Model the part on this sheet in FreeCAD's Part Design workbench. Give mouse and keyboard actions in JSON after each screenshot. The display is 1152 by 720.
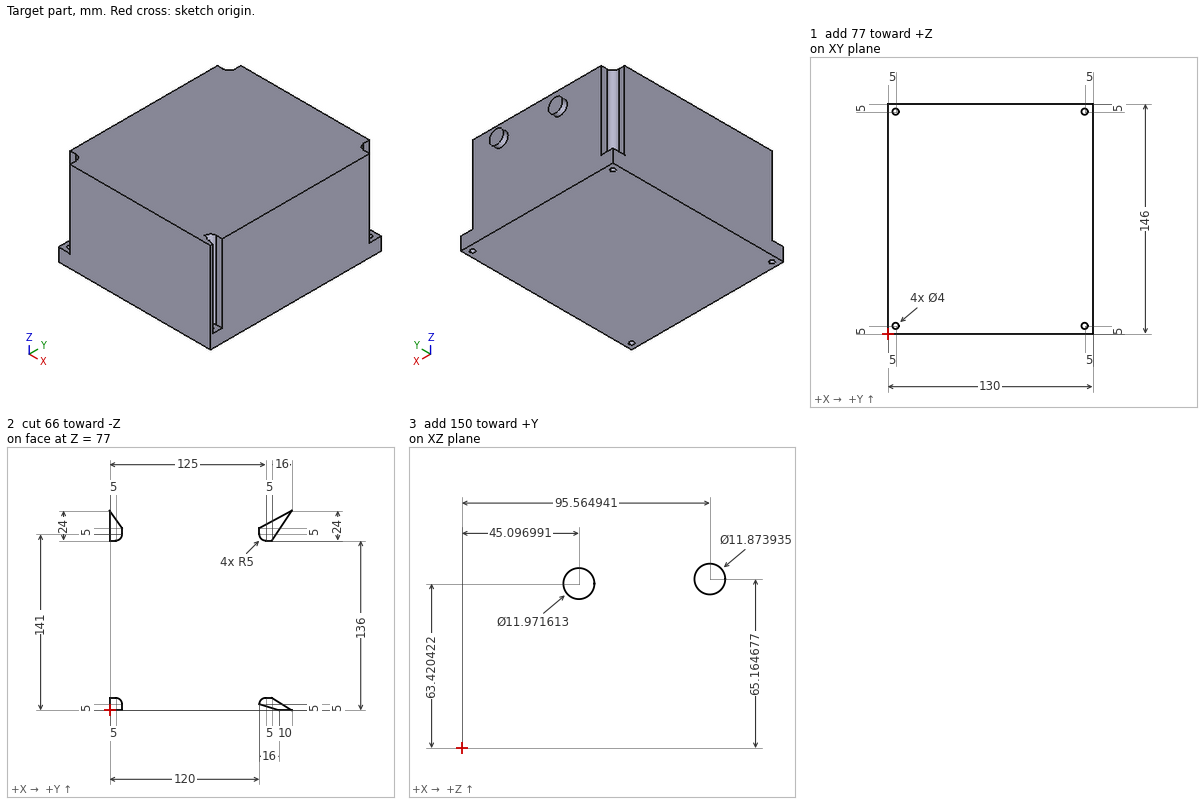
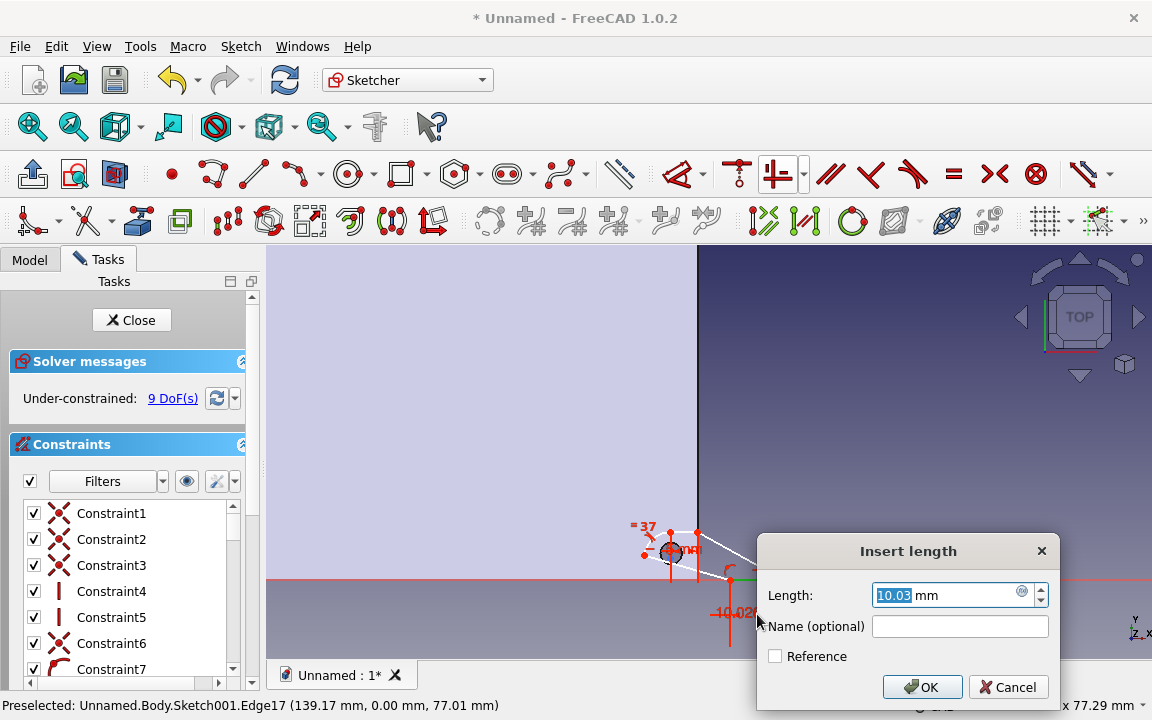
{"action": "type", "text": "10"}
{"action": "key", "text": "Return"}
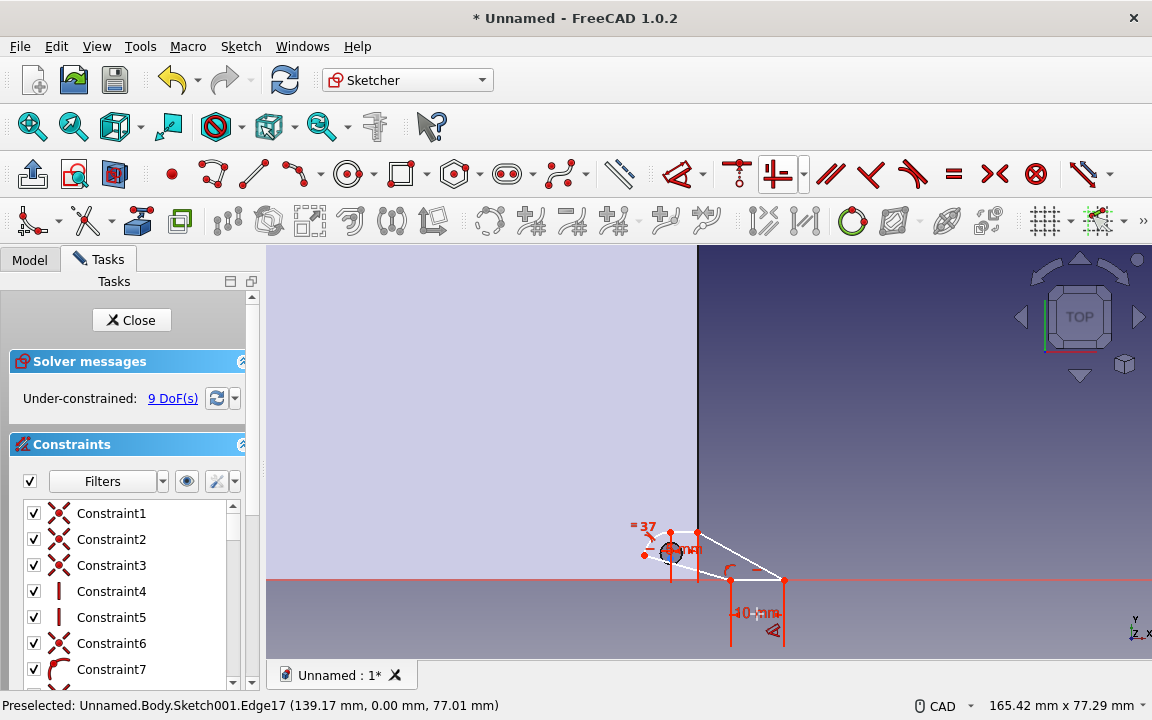
{"action": "scroll", "coordinate": [644, 555], "scroll_direction": "up", "scroll_amount": 2}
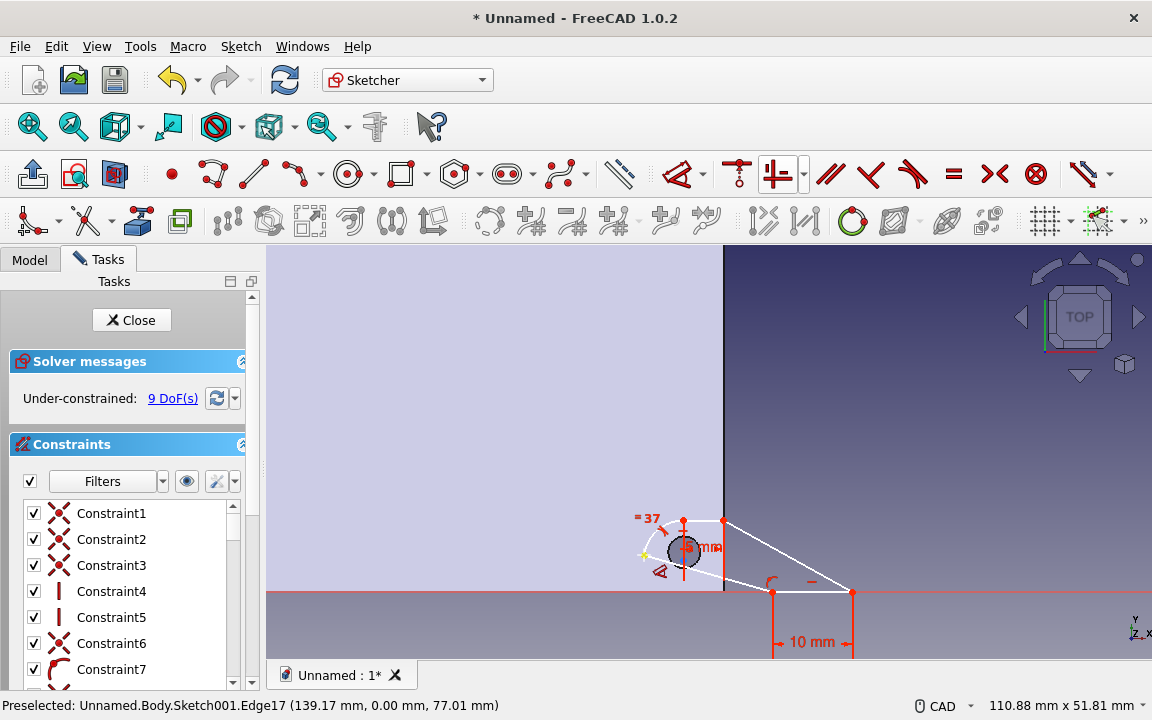
{"action": "left_click", "coordinate": [644, 555]}
{"action": "left_click", "coordinate": [774, 574]}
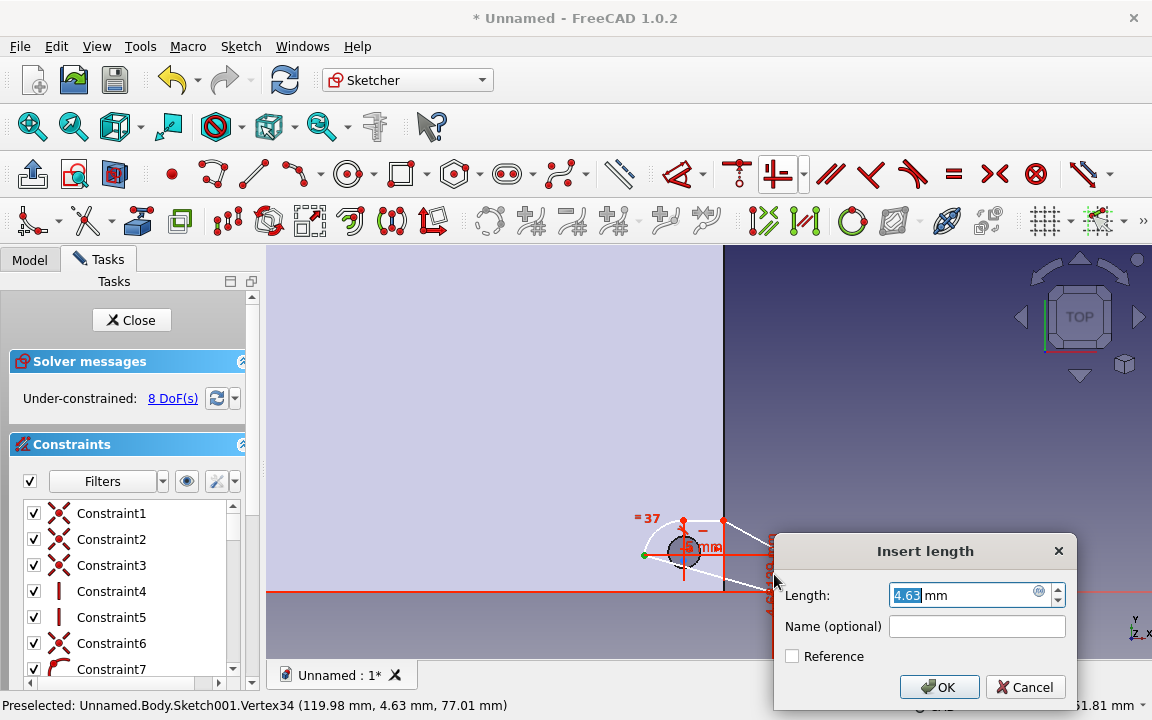
{"action": "type", "text": "5"}
{"action": "key", "text": "Return"}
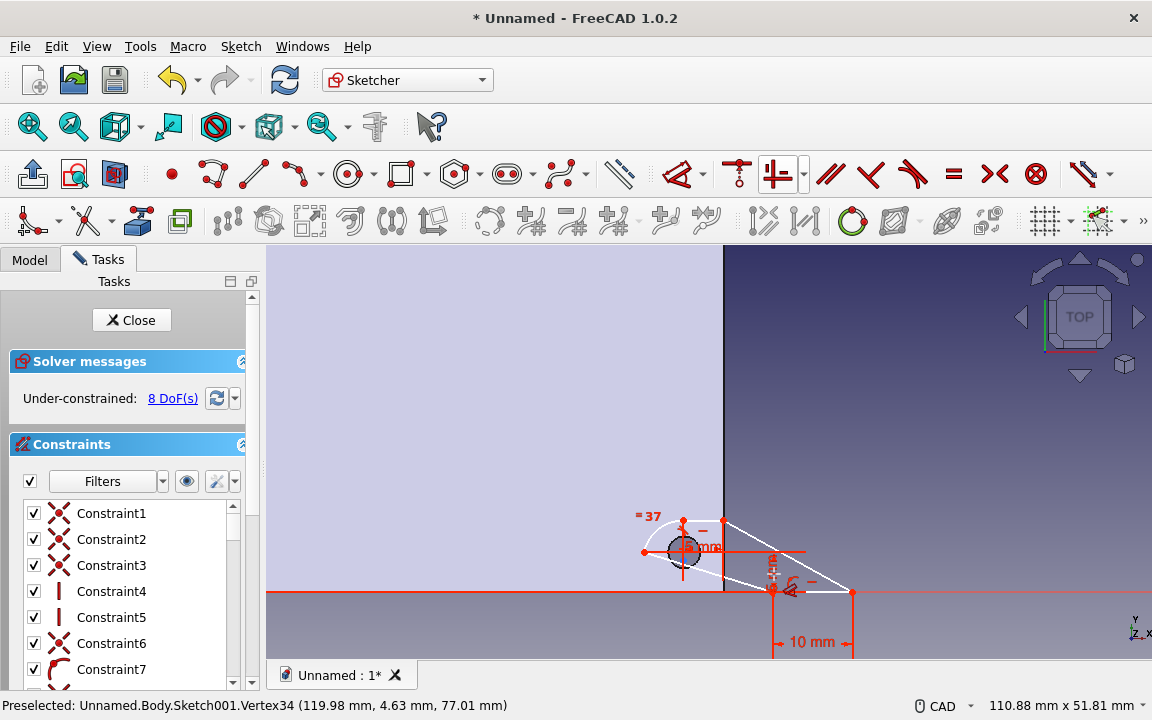
{"action": "left_click", "coordinate": [683, 561]}
{"action": "left_click", "coordinate": [863, 576]}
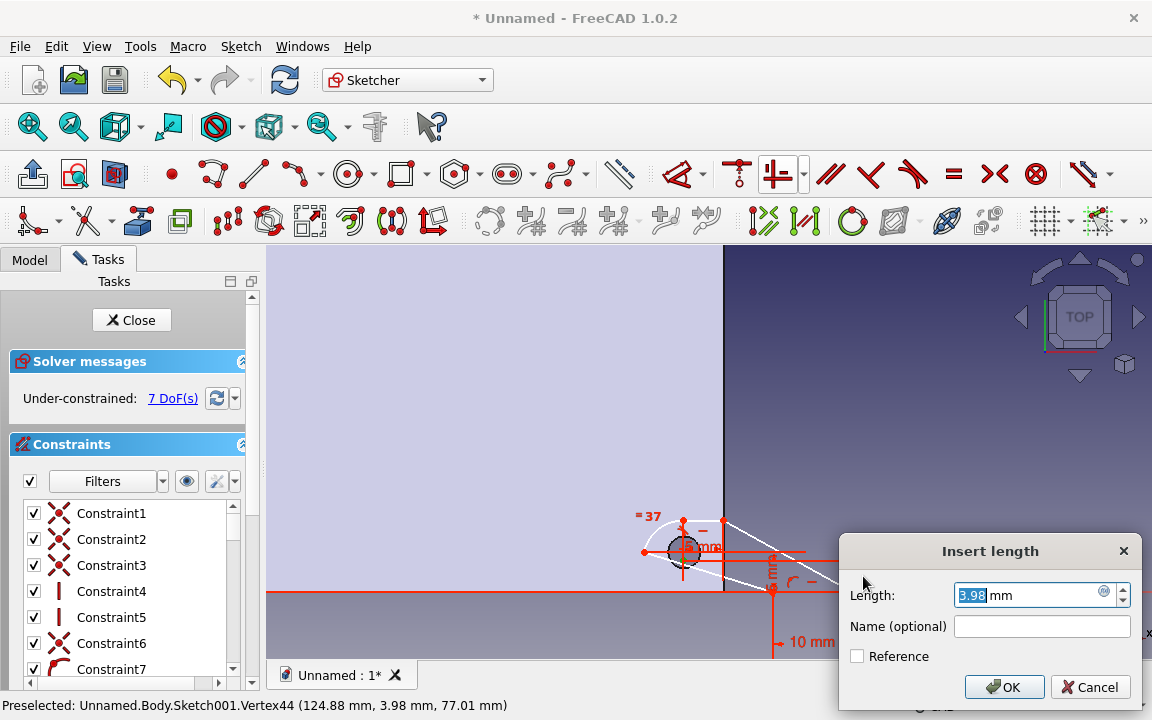
{"action": "type", "text": "5"}
{"action": "key", "text": "Return"}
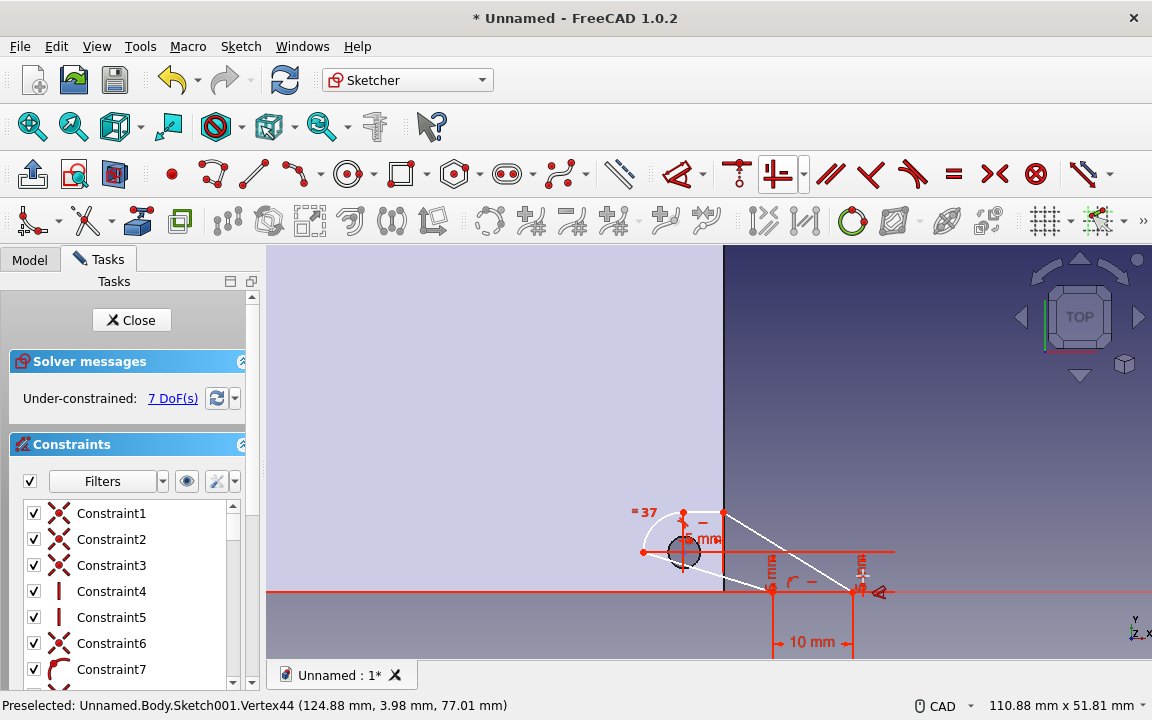
{"action": "scroll", "coordinate": [735, 578], "scroll_direction": "down", "scroll_amount": 8}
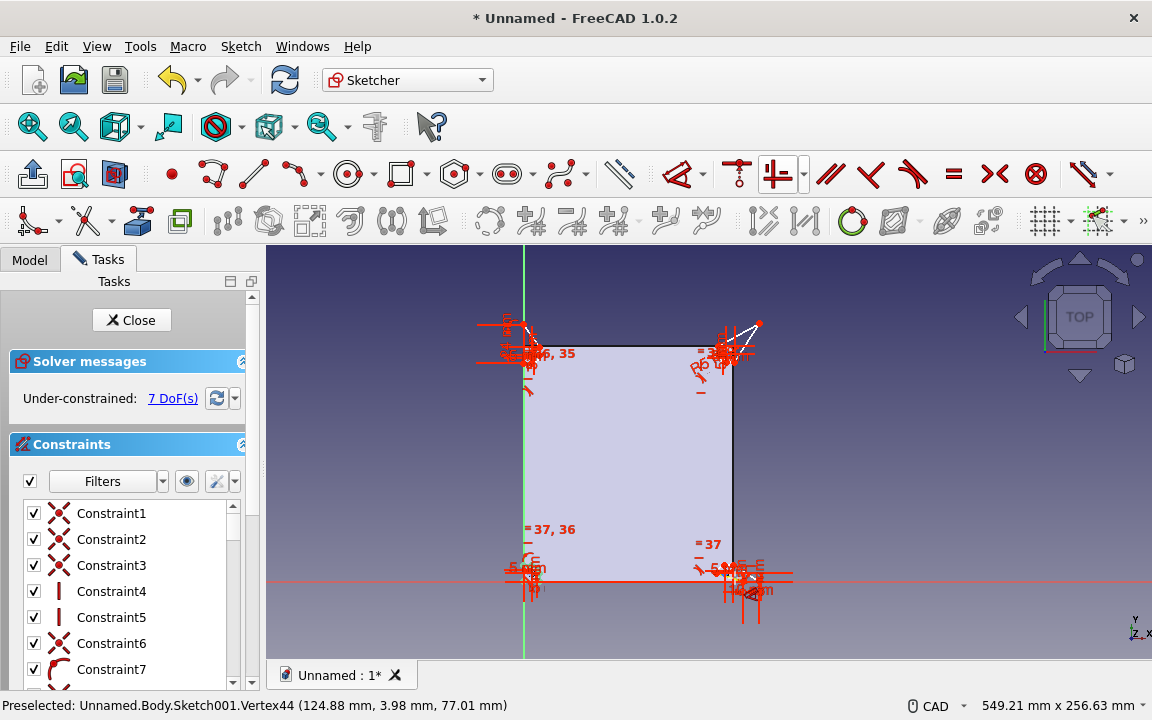
{"action": "scroll", "coordinate": [742, 351], "scroll_direction": "up", "scroll_amount": 3}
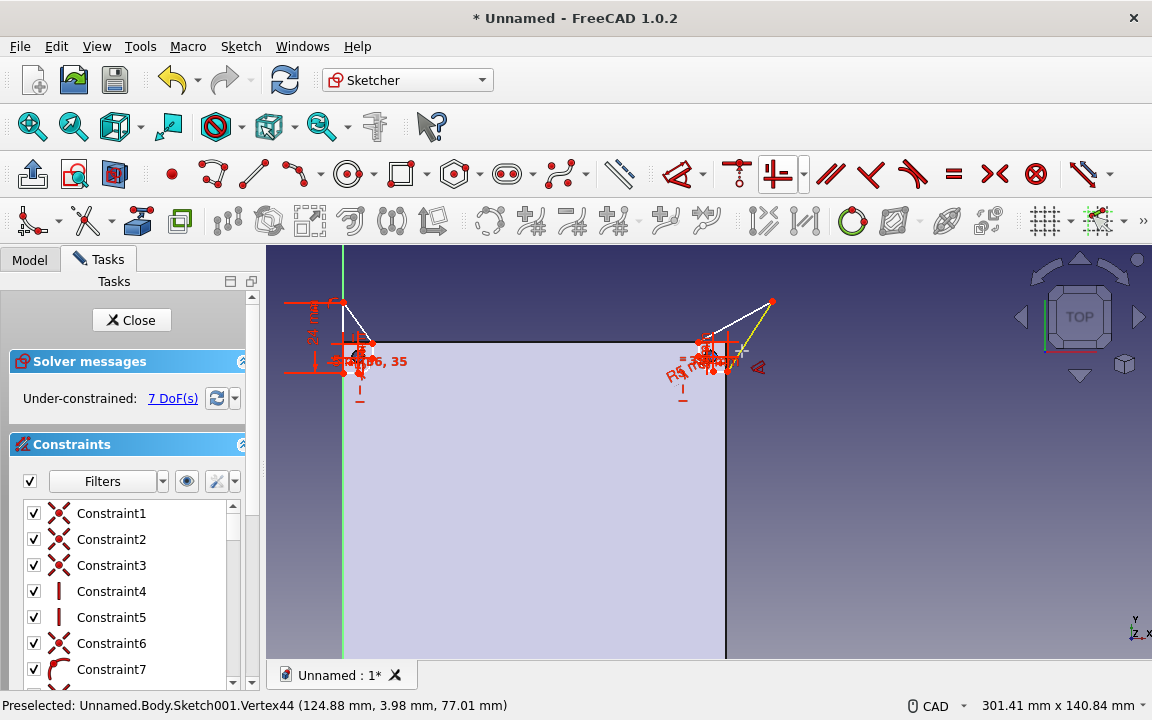
{"action": "left_click", "coordinate": [741, 351]}
{"action": "left_click", "coordinate": [750, 406]}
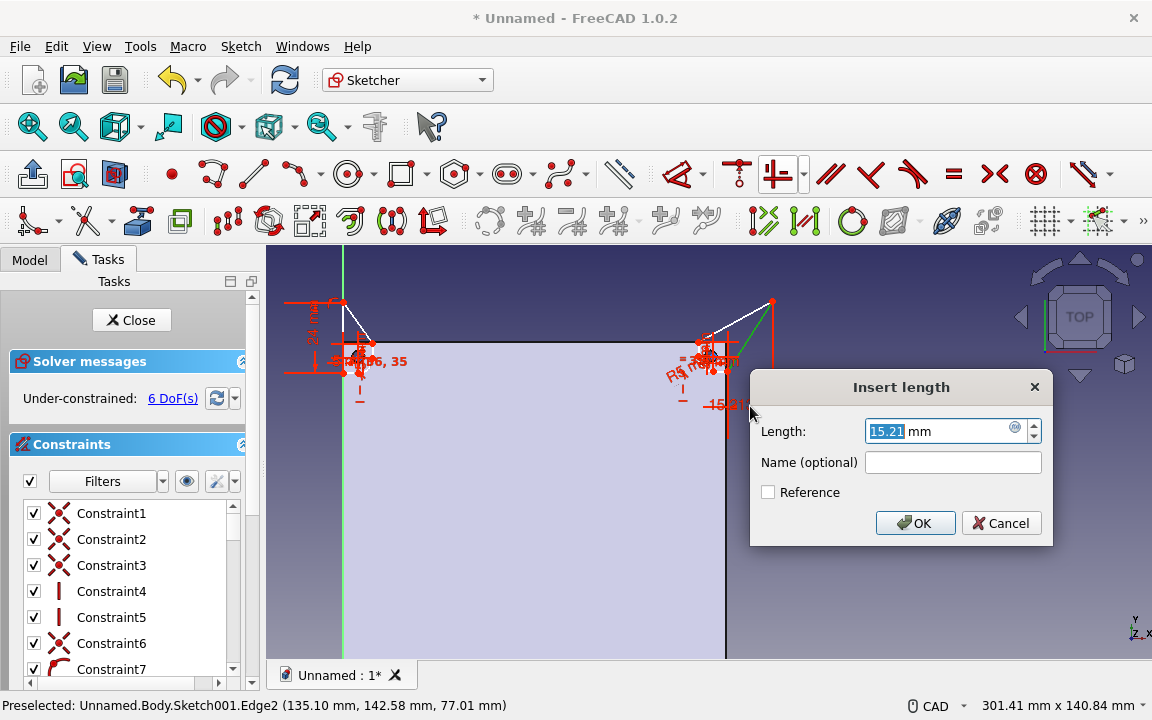
{"action": "type", "text": "16"}
{"action": "key", "text": "Return"}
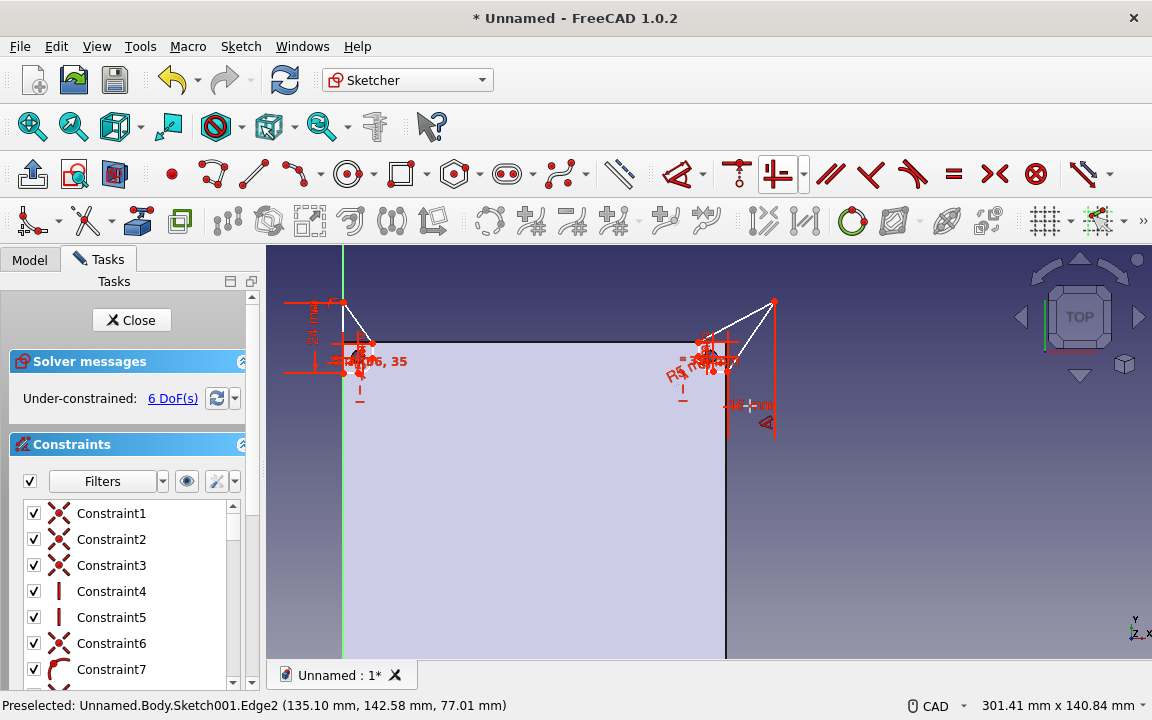
{"action": "left_click", "coordinate": [742, 351]}
{"action": "left_click", "coordinate": [809, 337]}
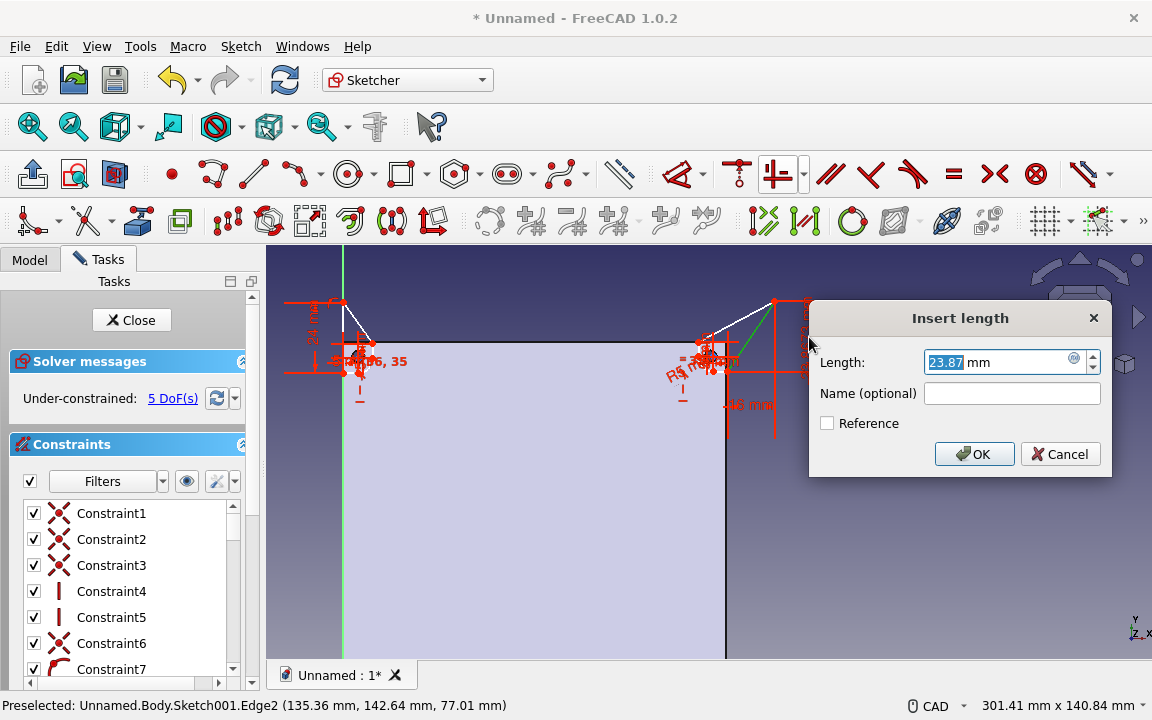
{"action": "type", "text": "24"}
{"action": "key", "text": "Return"}